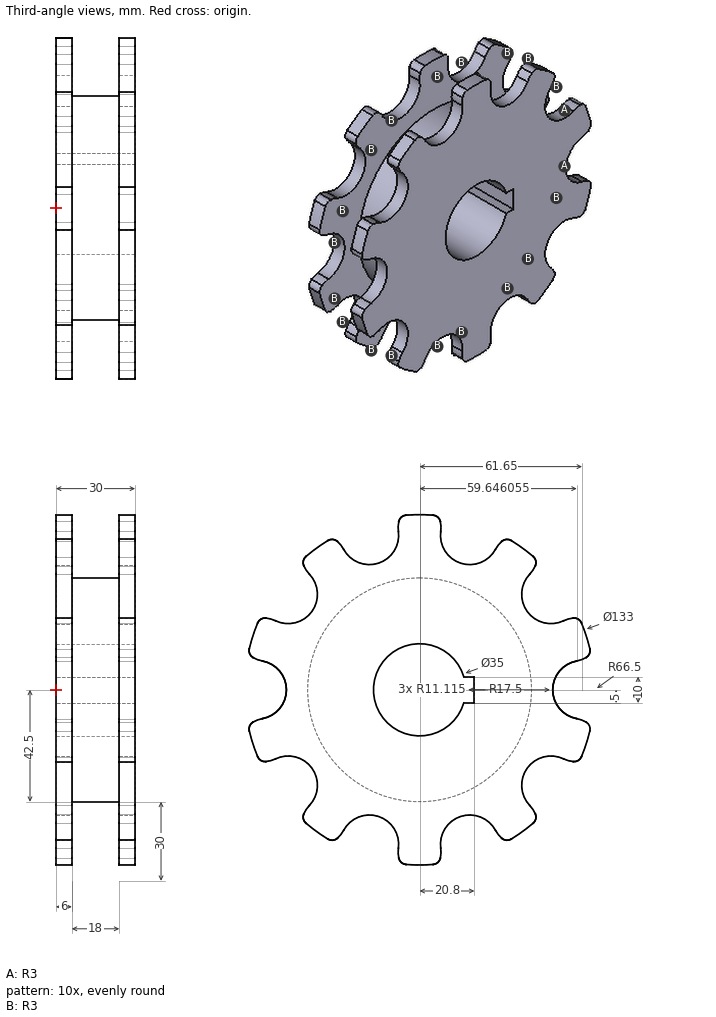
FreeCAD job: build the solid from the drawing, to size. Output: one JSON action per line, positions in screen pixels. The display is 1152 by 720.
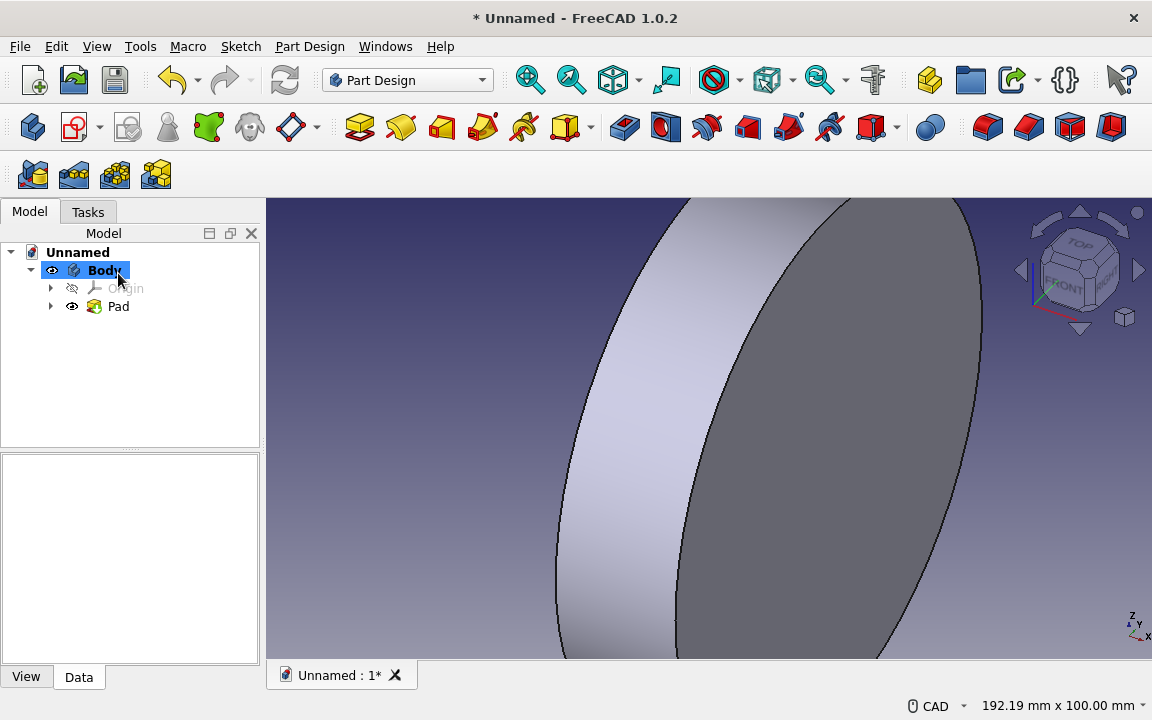
{"action": "left_click", "coordinate": [531, 80]}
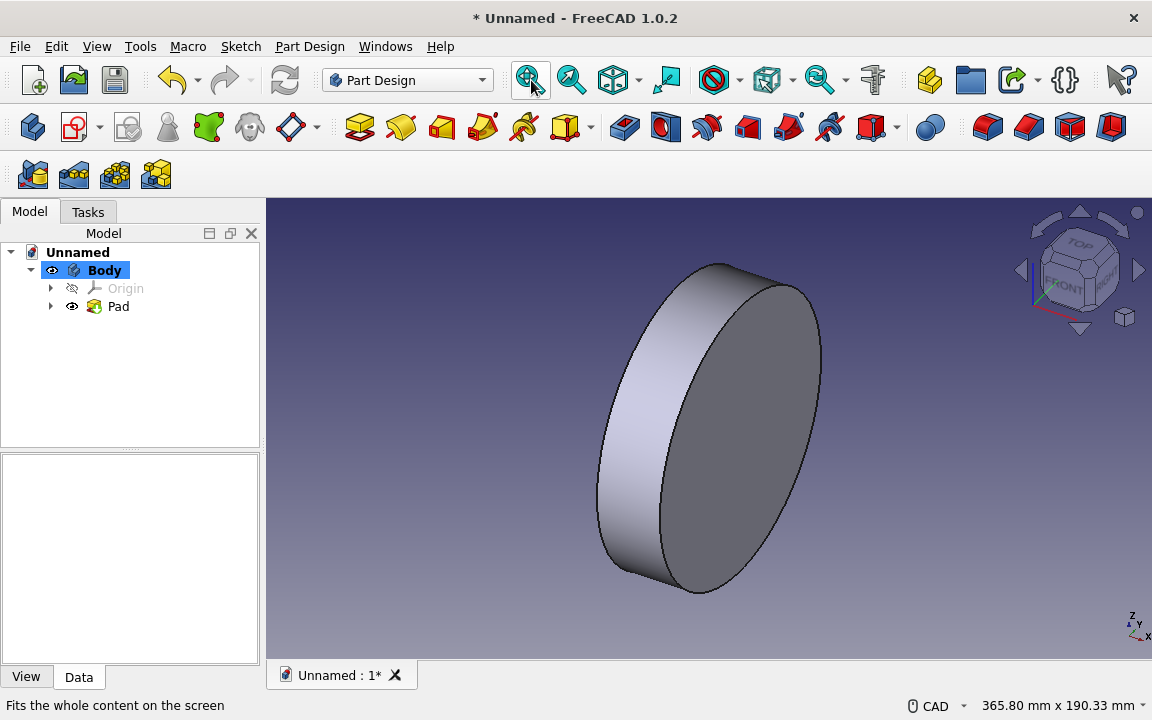
{"action": "left_click", "coordinate": [740, 438]}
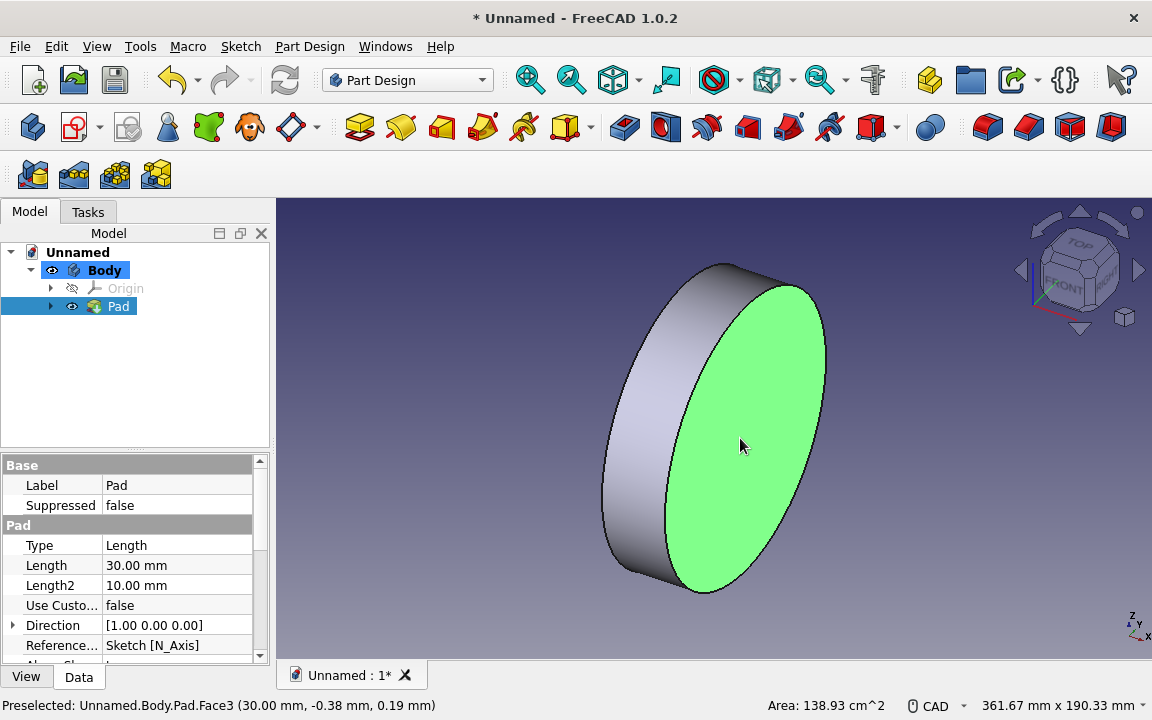
{"action": "left_click", "coordinate": [74, 128]}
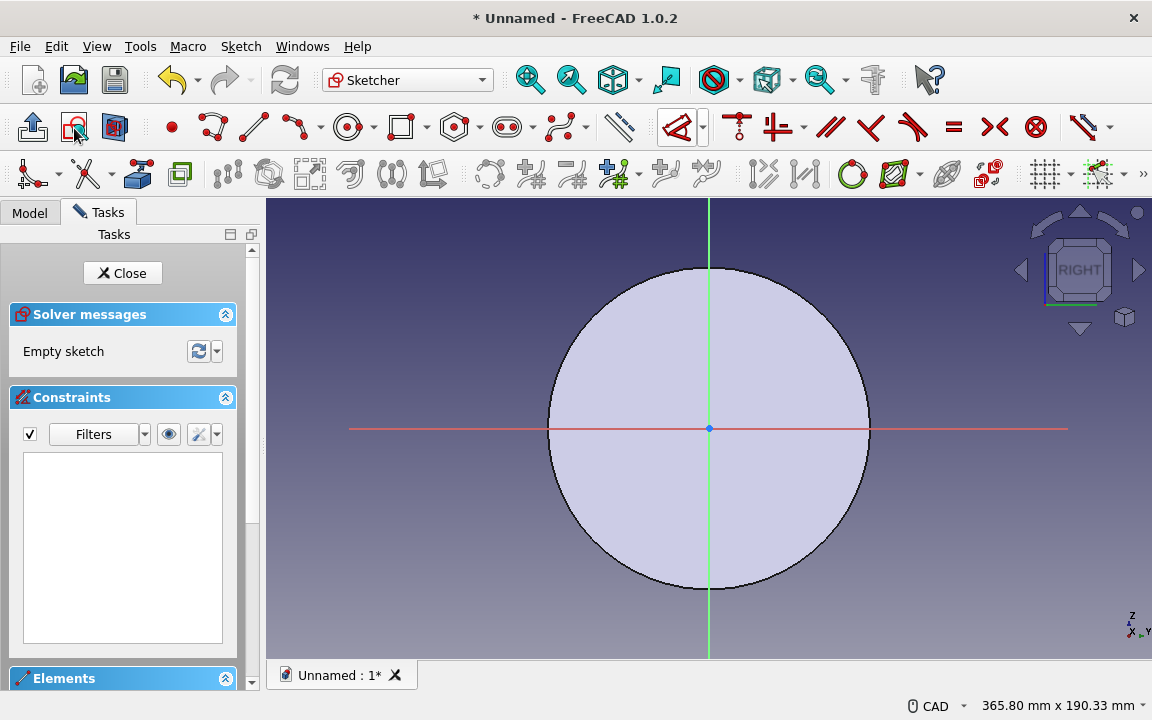
{"action": "scroll", "coordinate": [739, 428], "scroll_direction": "up", "scroll_amount": 6}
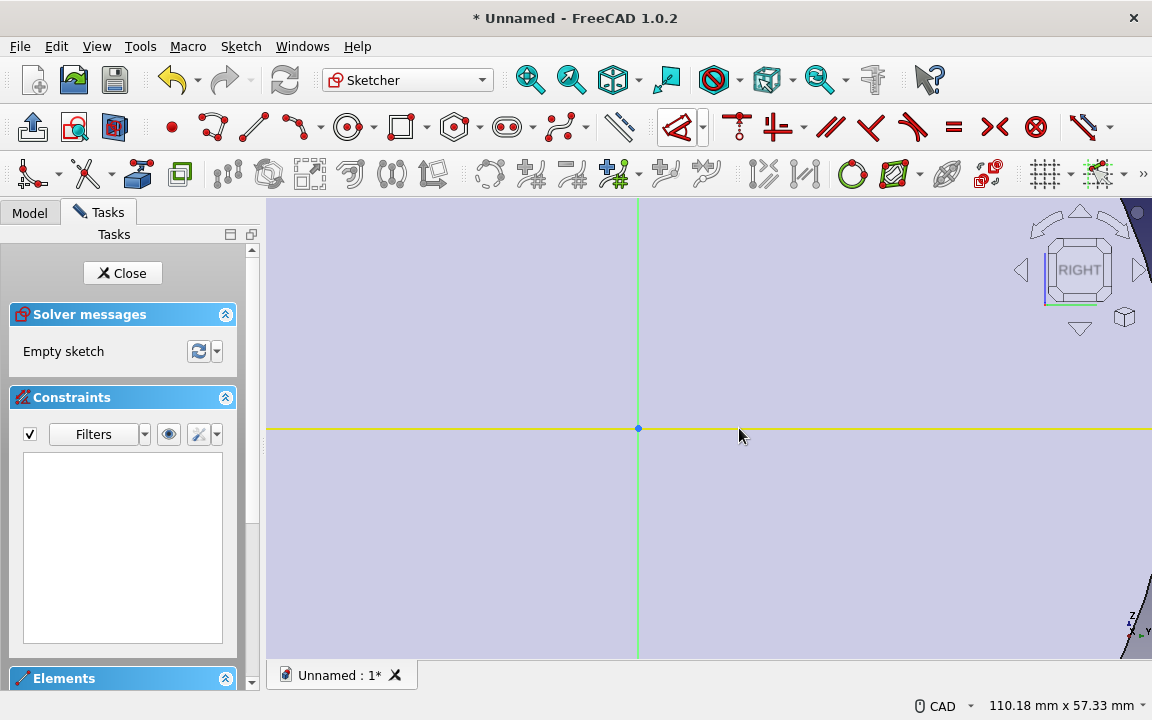
{"action": "left_click", "coordinate": [348, 128]}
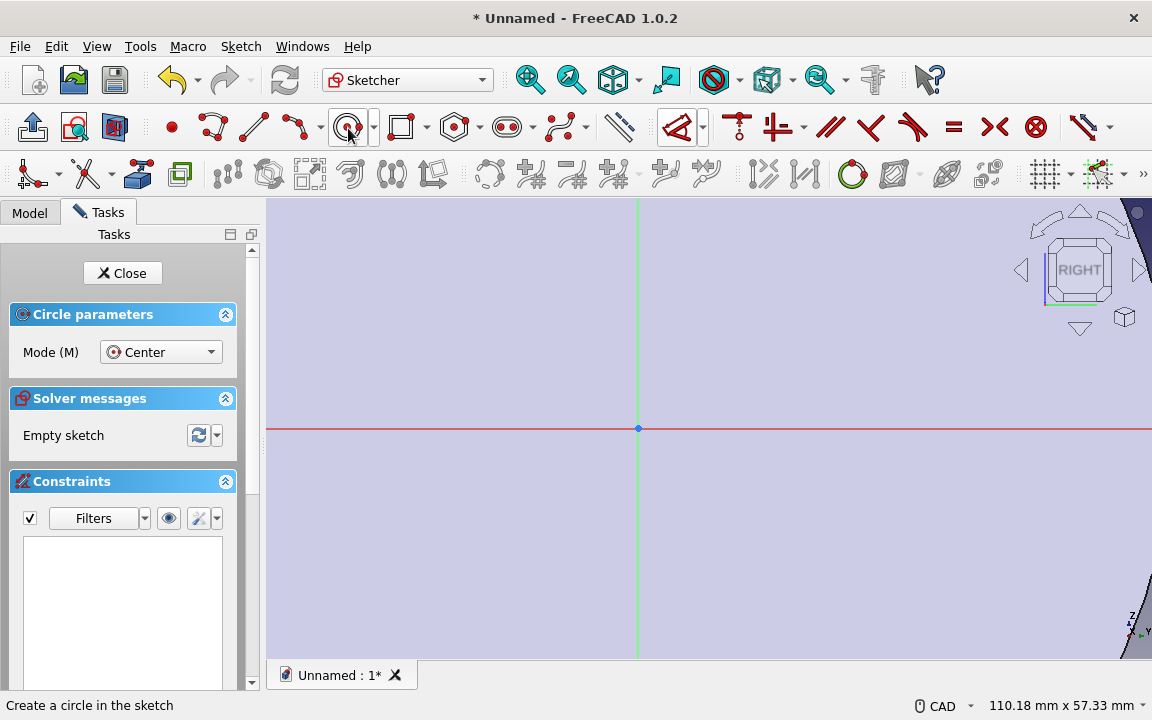
{"action": "left_click", "coordinate": [638, 428]}
{"action": "mouse_move", "coordinate": [738, 329]}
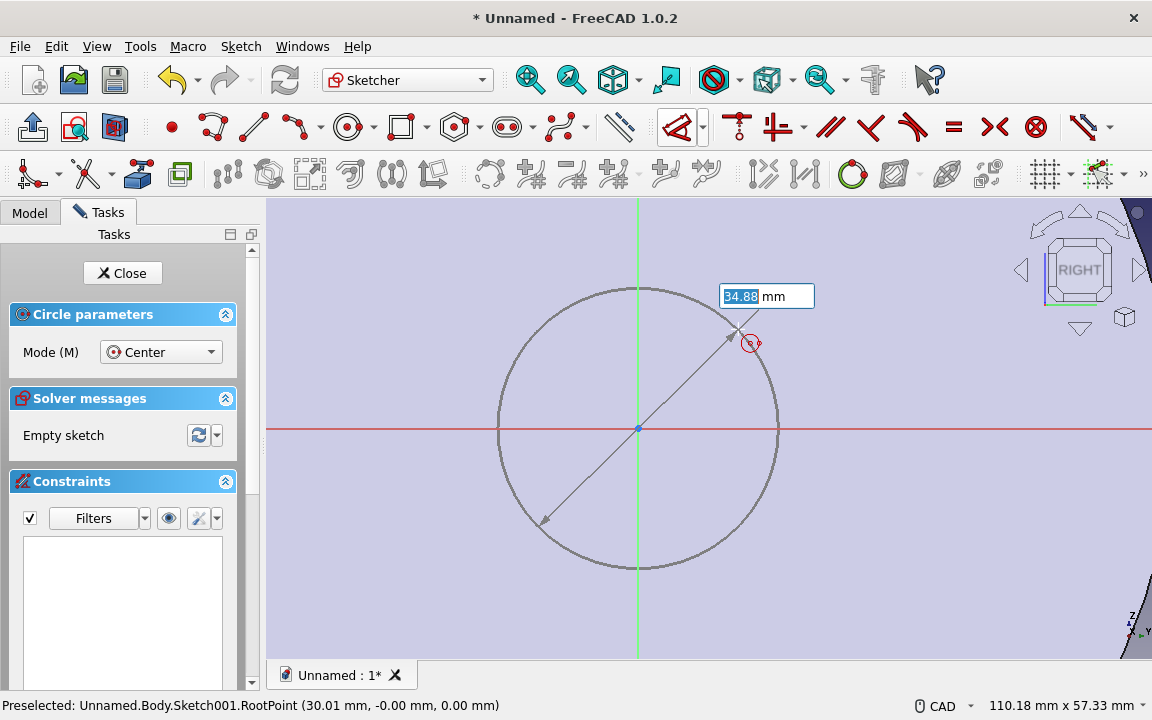
{"action": "type", "text": "35"}
{"action": "key", "text": "Return"}
{"action": "key", "text": "Escape"}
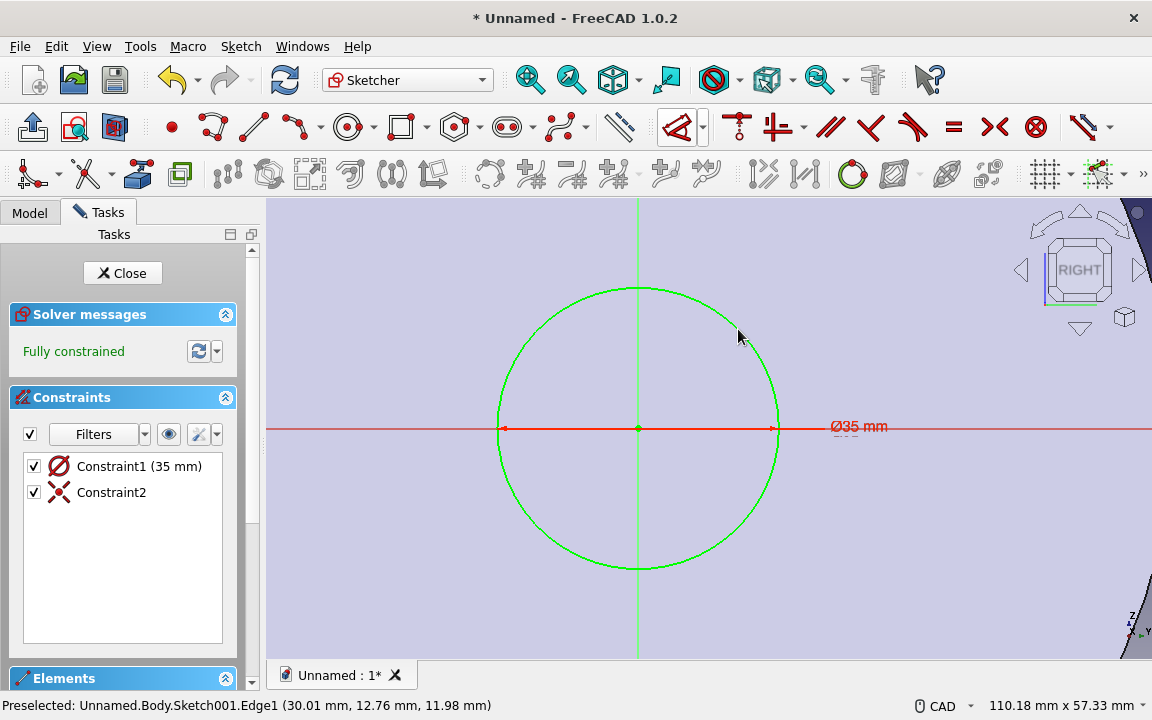
{"action": "left_click", "coordinate": [123, 273]}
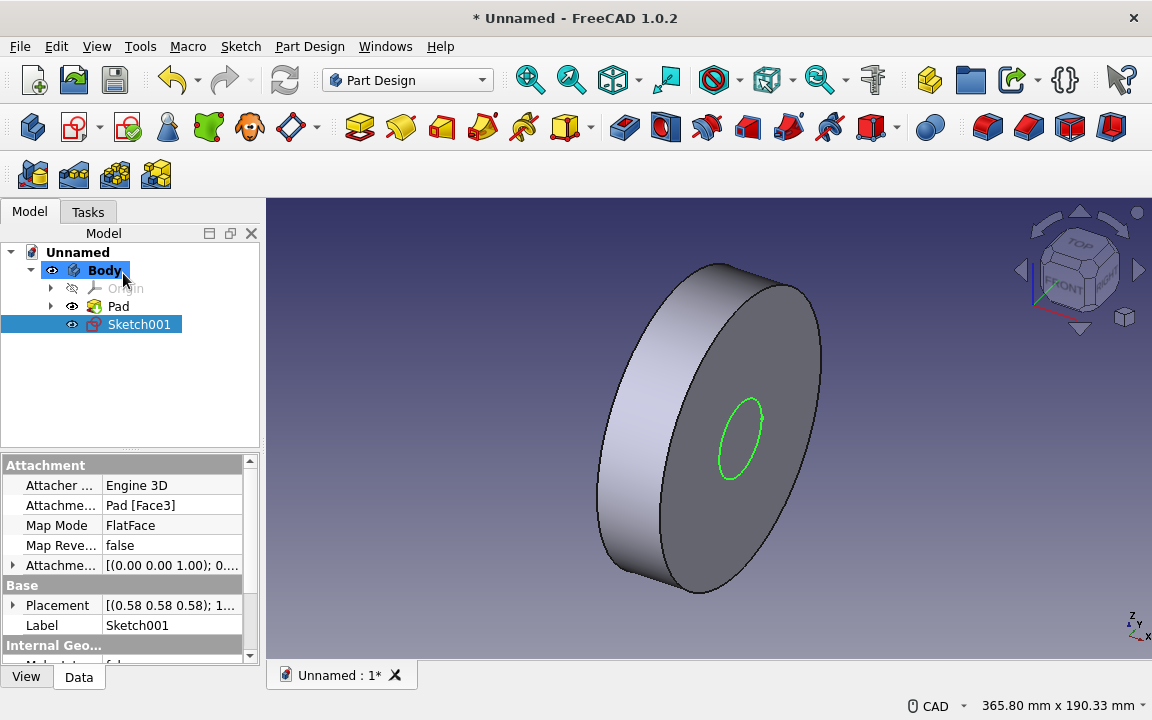
{"action": "left_click", "coordinate": [625, 128]}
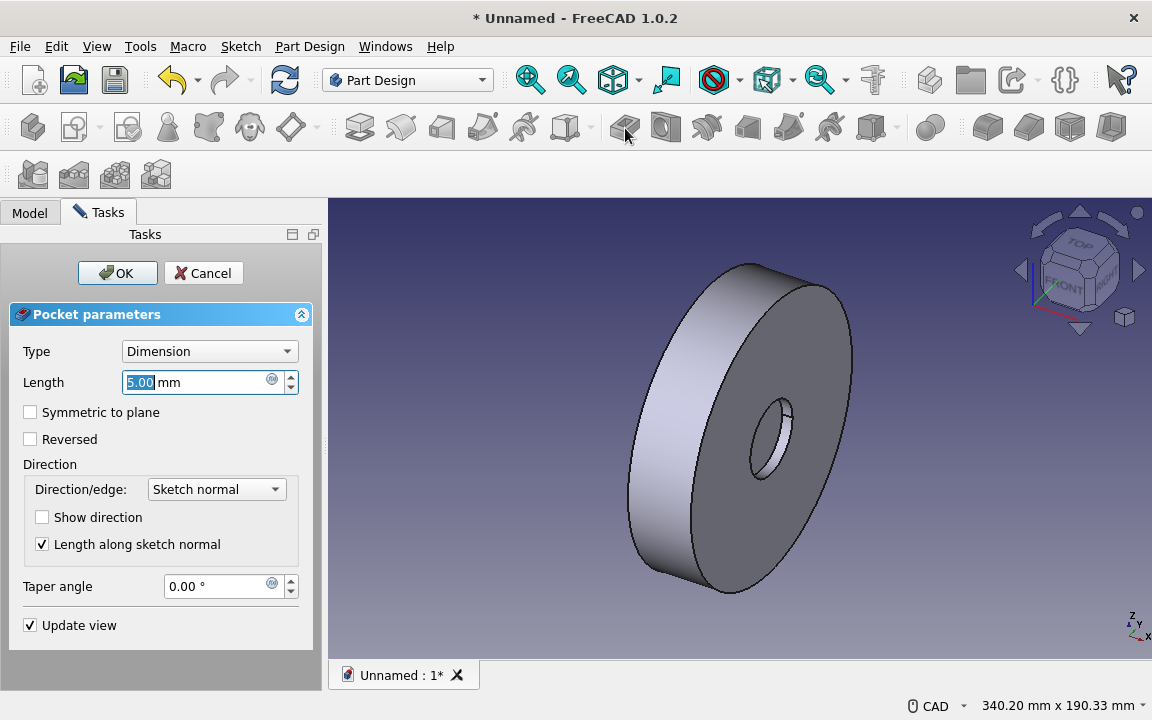
{"action": "left_click", "coordinate": [210, 352]}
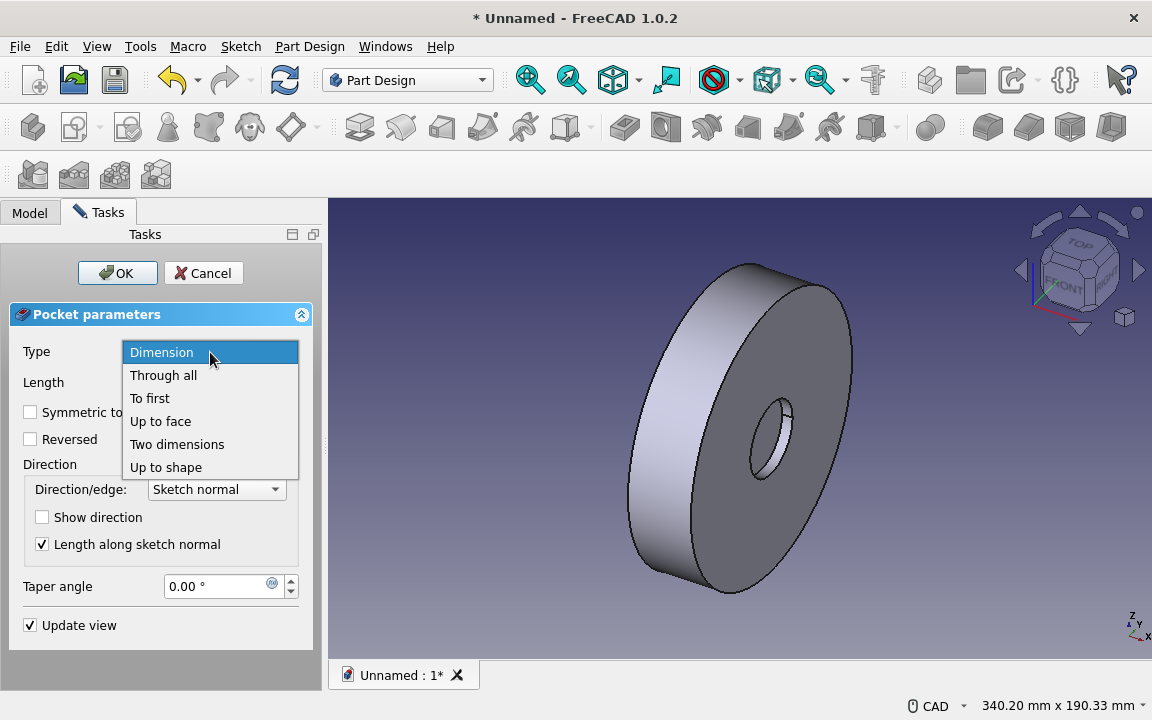
{"action": "left_click", "coordinate": [208, 376]}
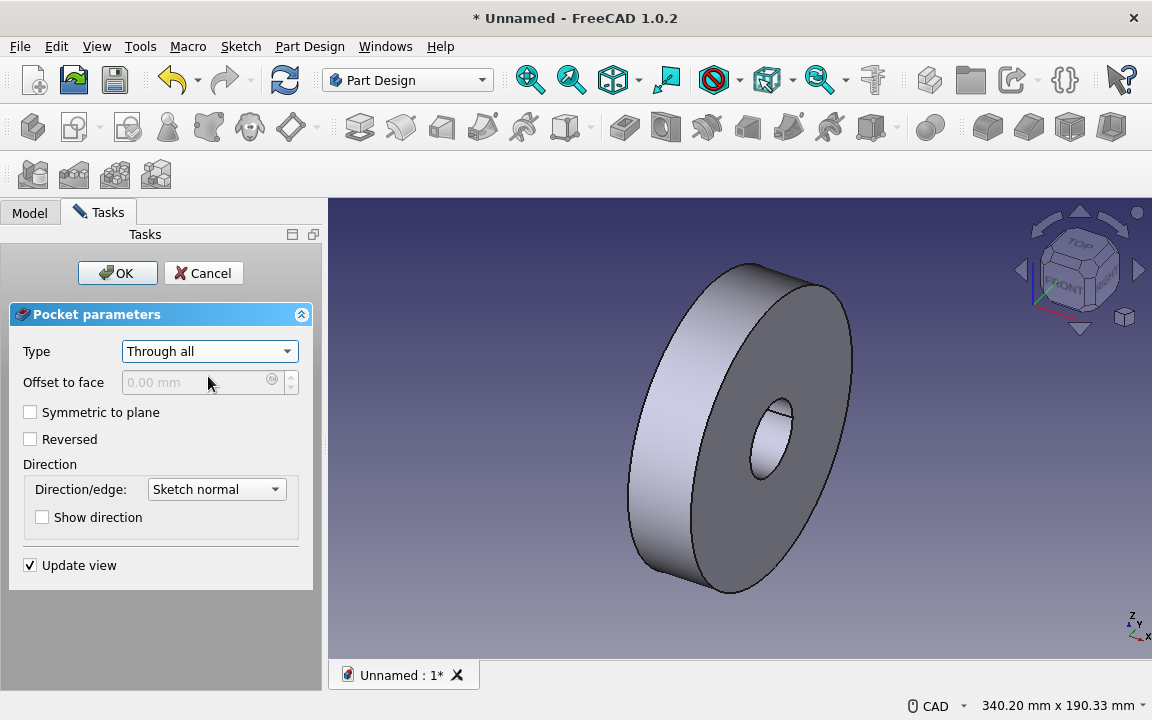
{"action": "left_click", "coordinate": [118, 273]}